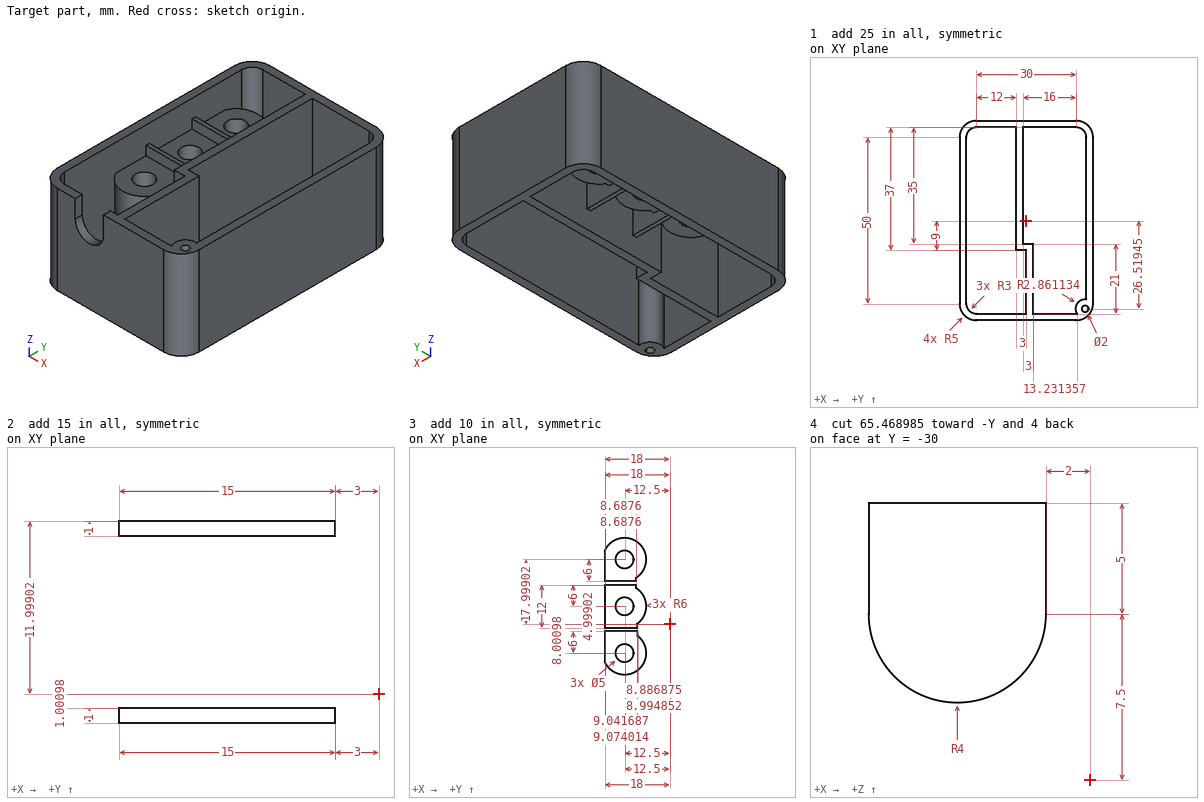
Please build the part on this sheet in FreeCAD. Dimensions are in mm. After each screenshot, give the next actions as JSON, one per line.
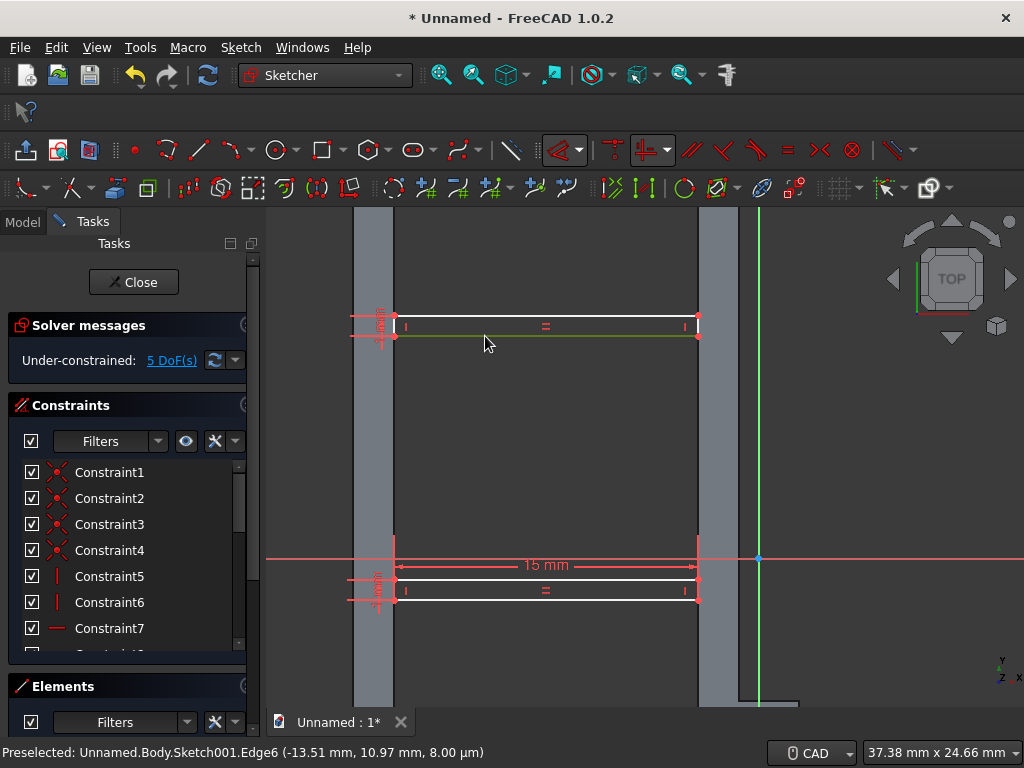
{"action": "left_click", "coordinate": [582, 150]}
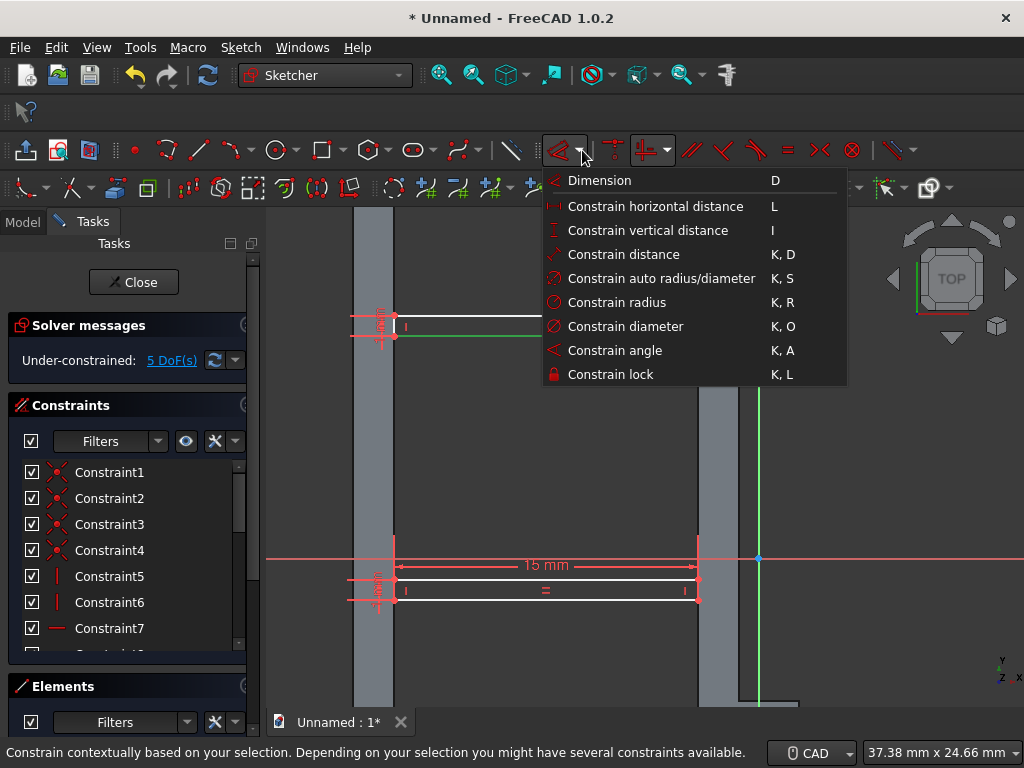
{"action": "left_click", "coordinate": [695, 206]}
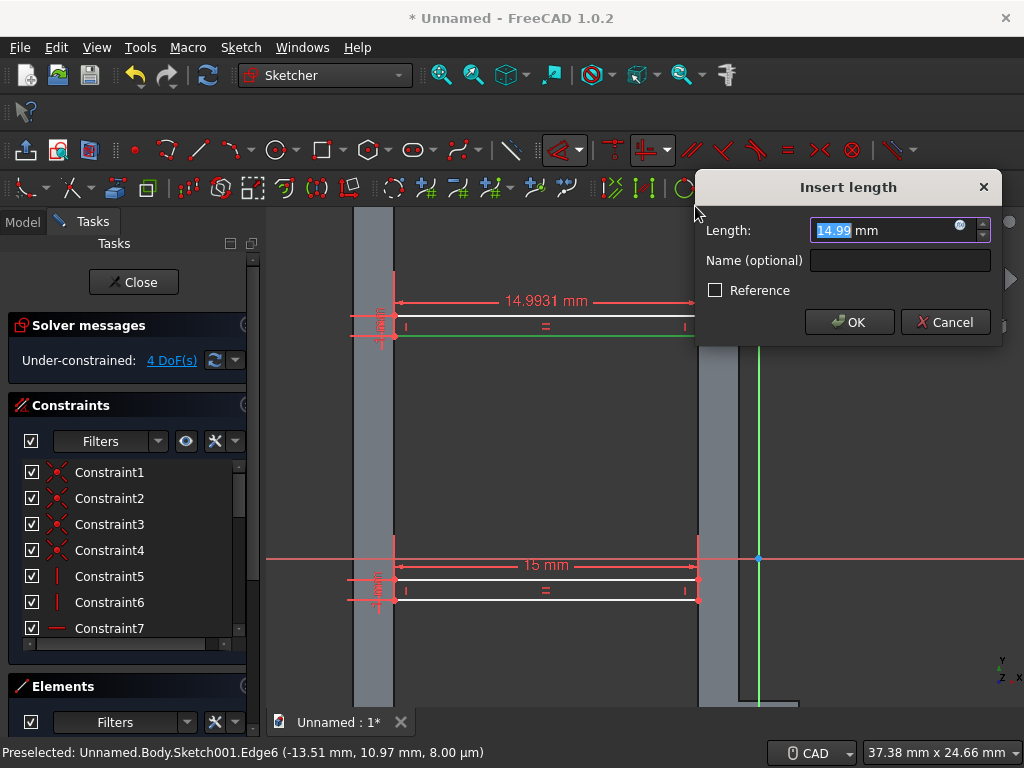
{"action": "type", "text": "15"}
{"action": "key", "text": "Return"}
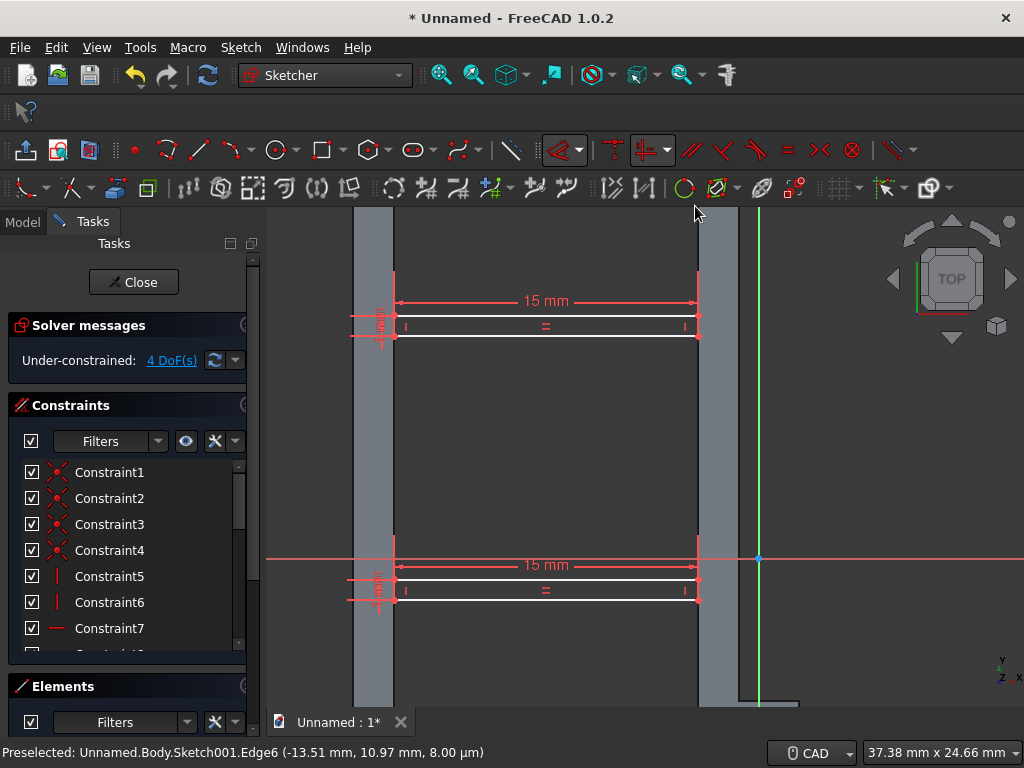
{"action": "left_click", "coordinate": [698, 600]}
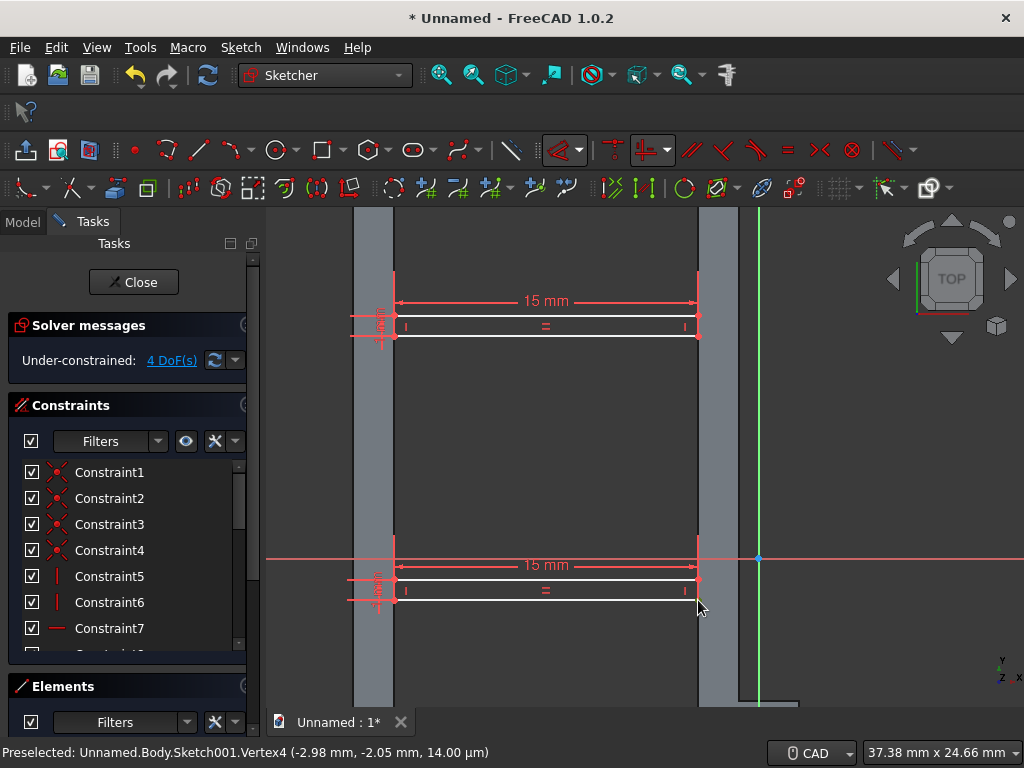
{"action": "left_click", "coordinate": [582, 150]}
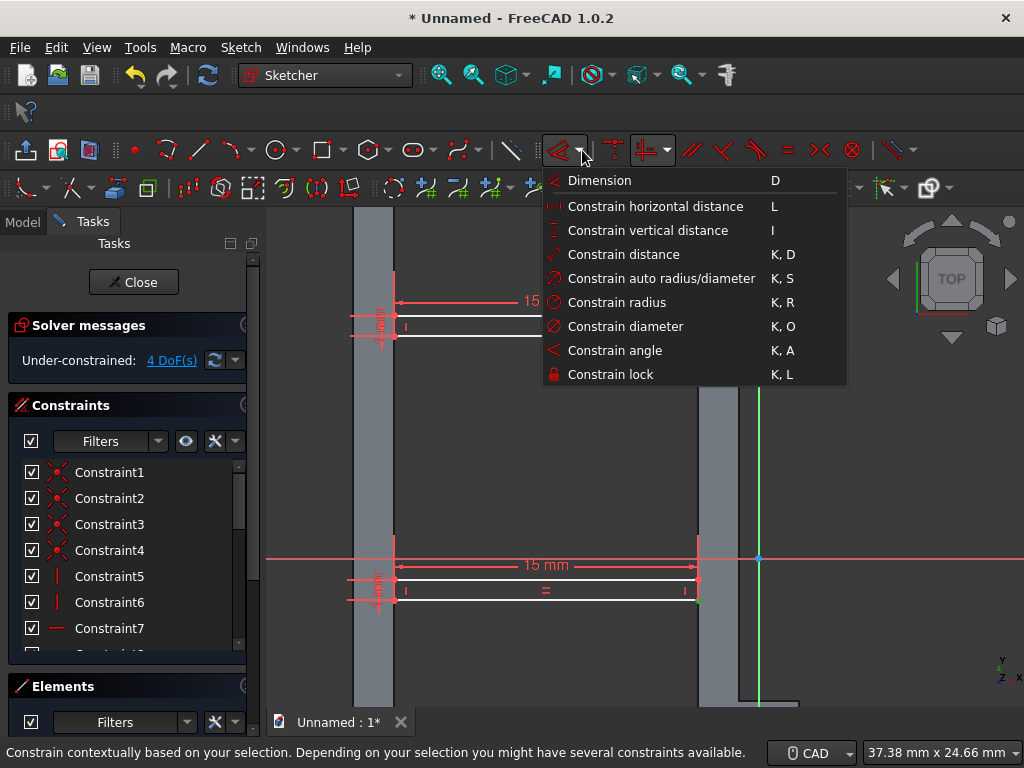
{"action": "left_click", "coordinate": [695, 206]}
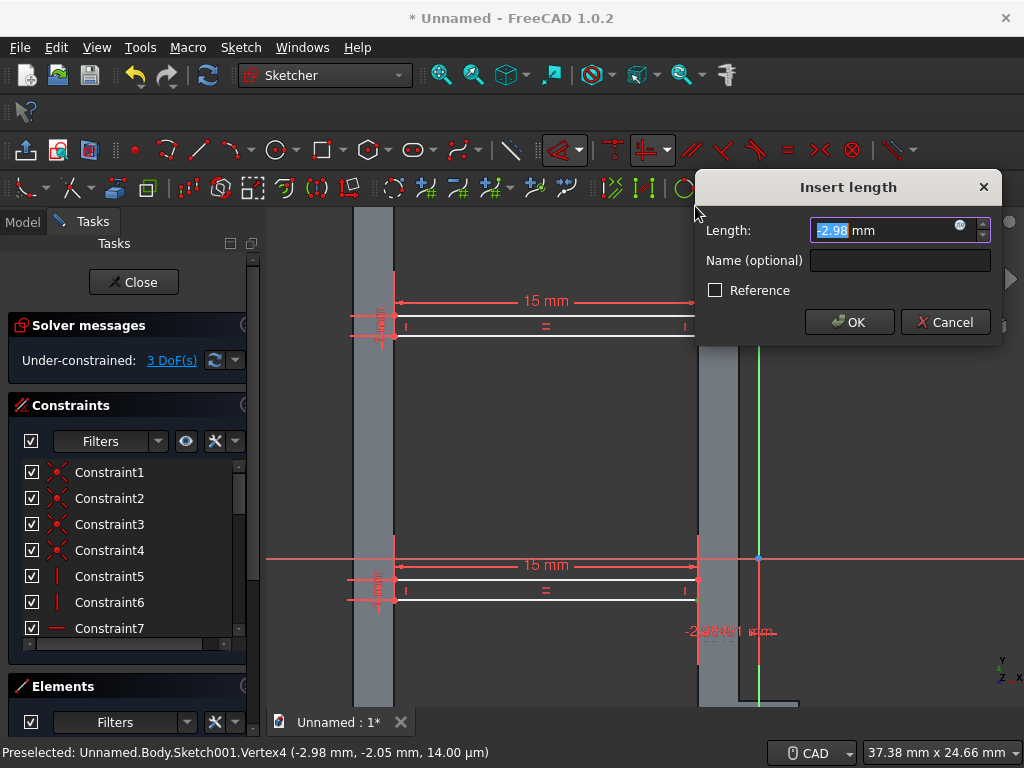
{"action": "type", "text": "-3"}
{"action": "key", "text": "Return"}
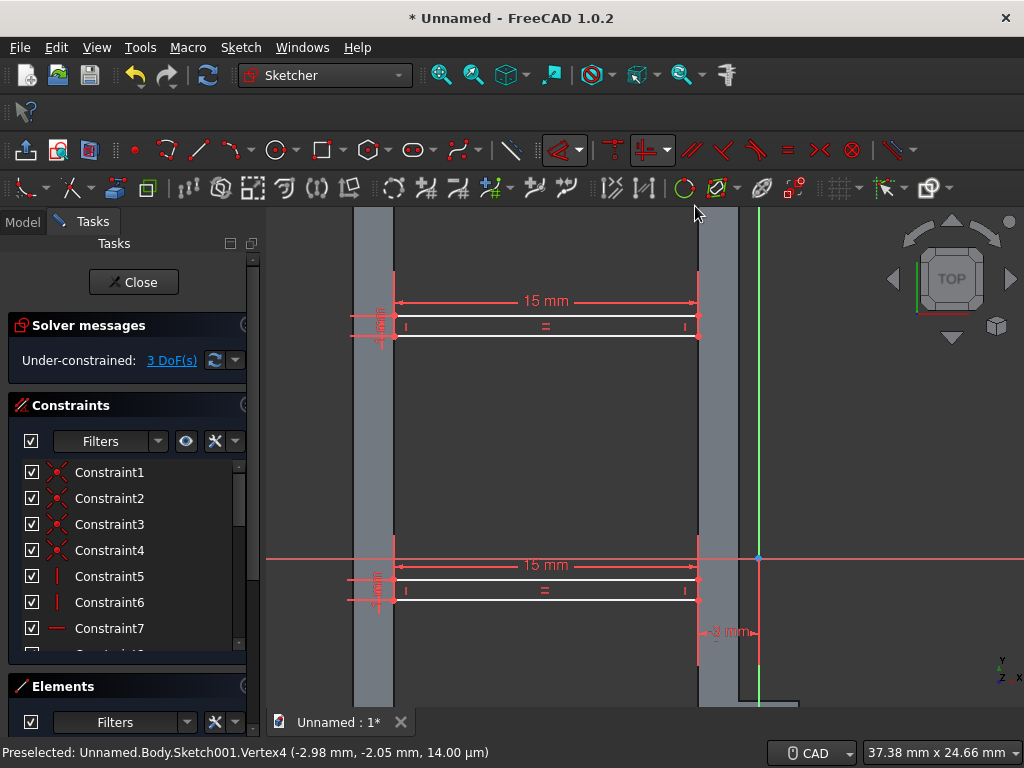
{"action": "left_click", "coordinate": [698, 336]}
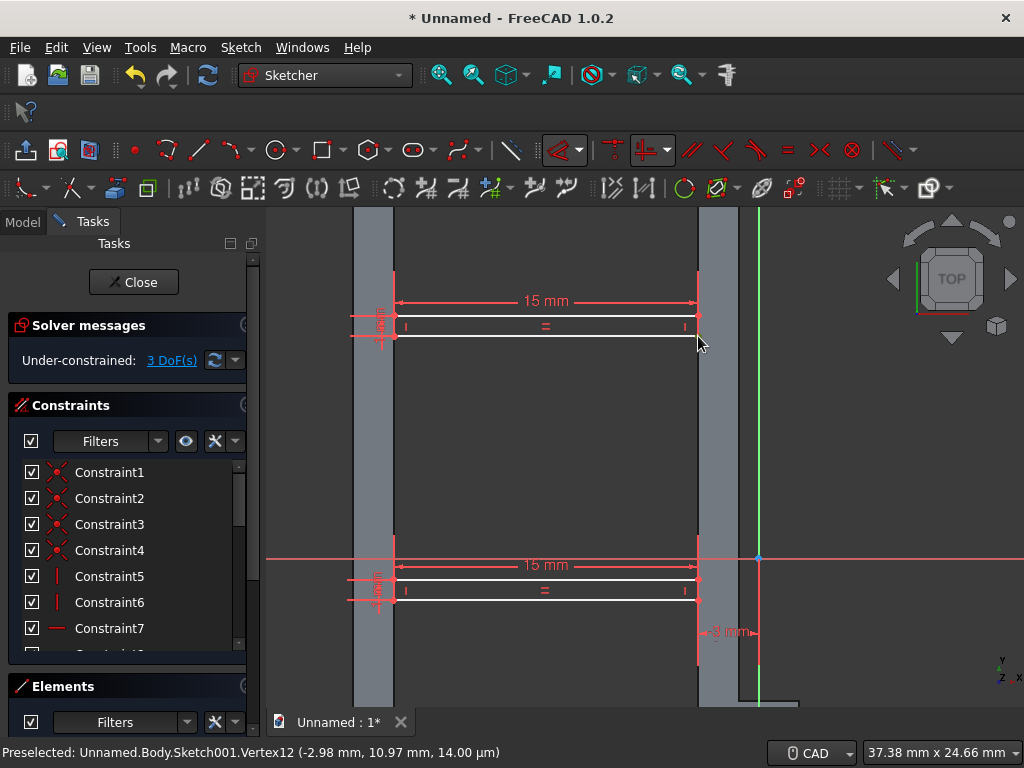
{"action": "left_click", "coordinate": [582, 150]}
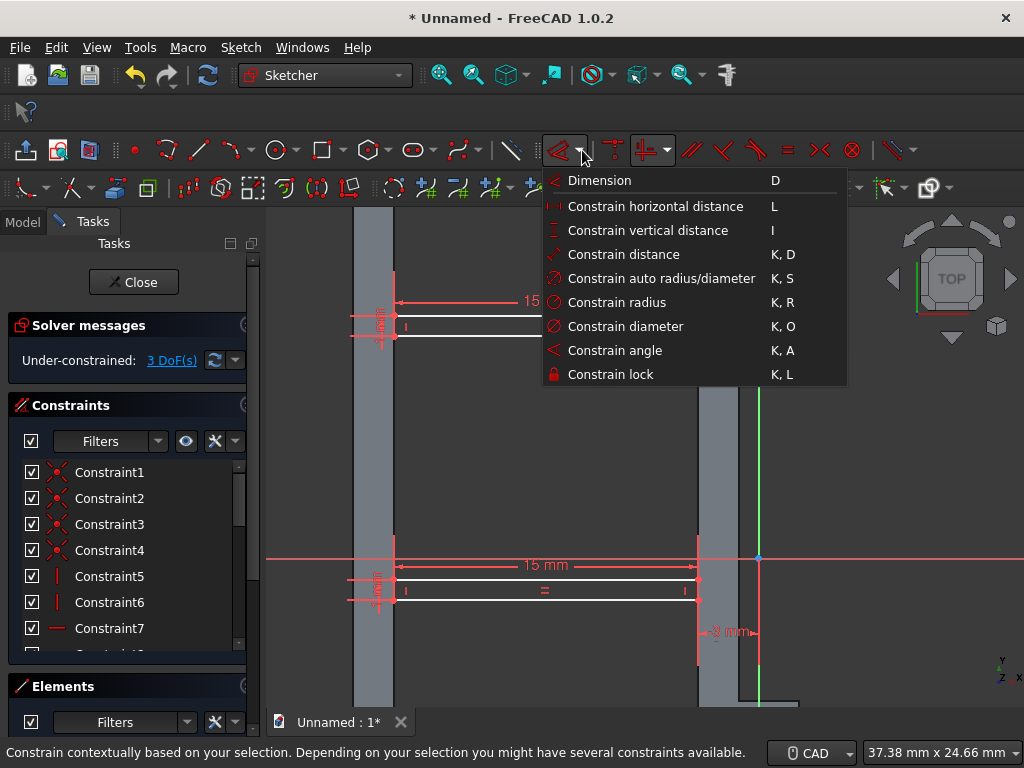
{"action": "left_click", "coordinate": [695, 206]}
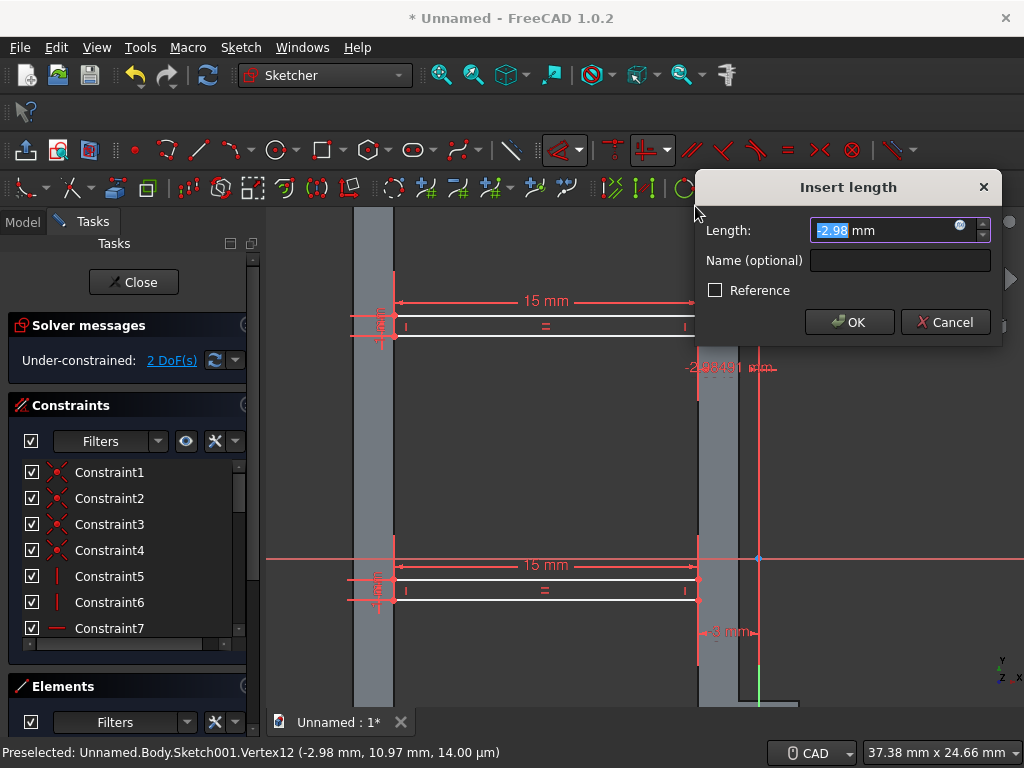
{"action": "type", "text": "-3"}
{"action": "key", "text": "Return"}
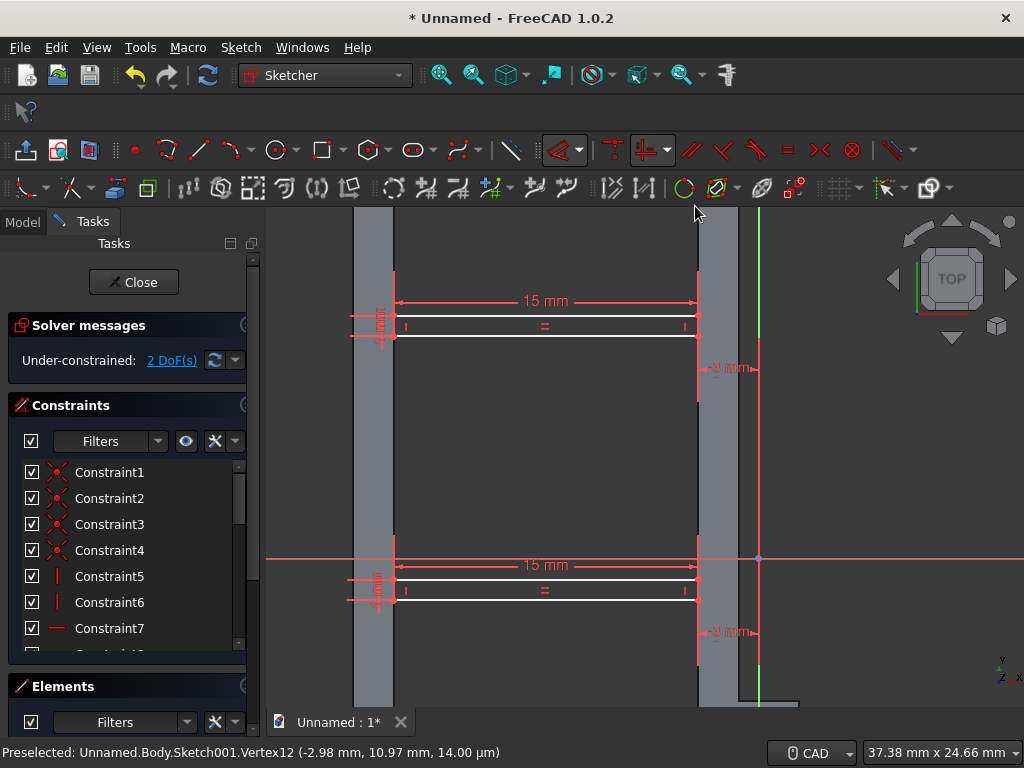
{"action": "scroll", "coordinate": [394, 580], "scroll_direction": "up", "scroll_amount": 4}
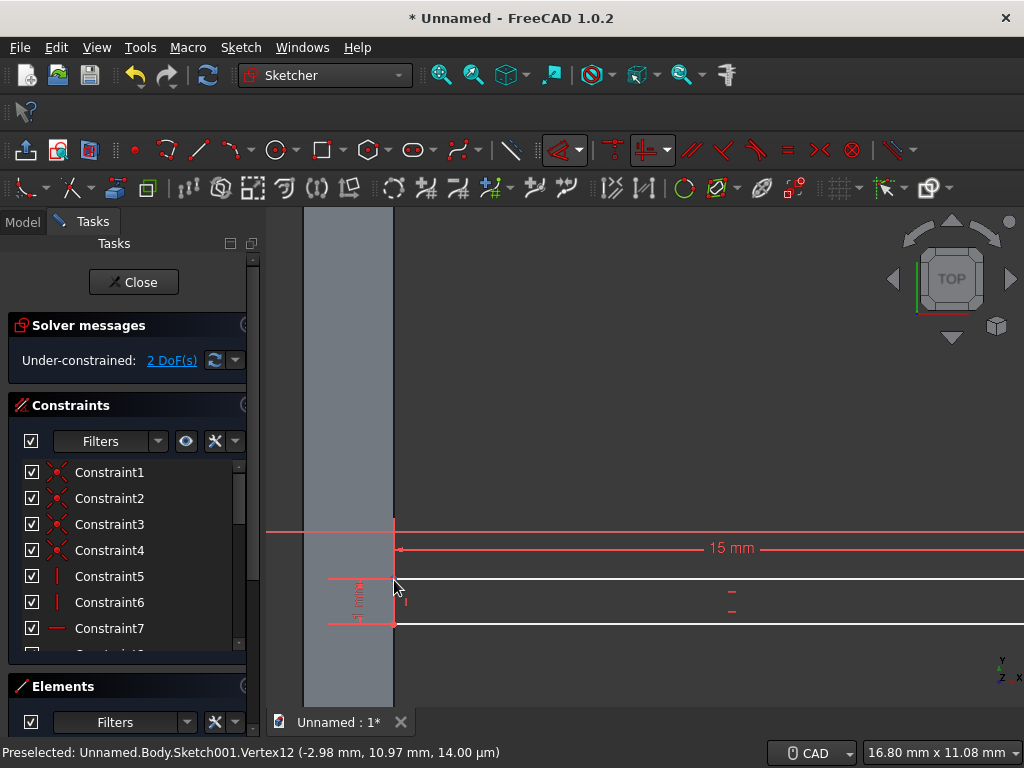
{"action": "left_click", "coordinate": [394, 579]}